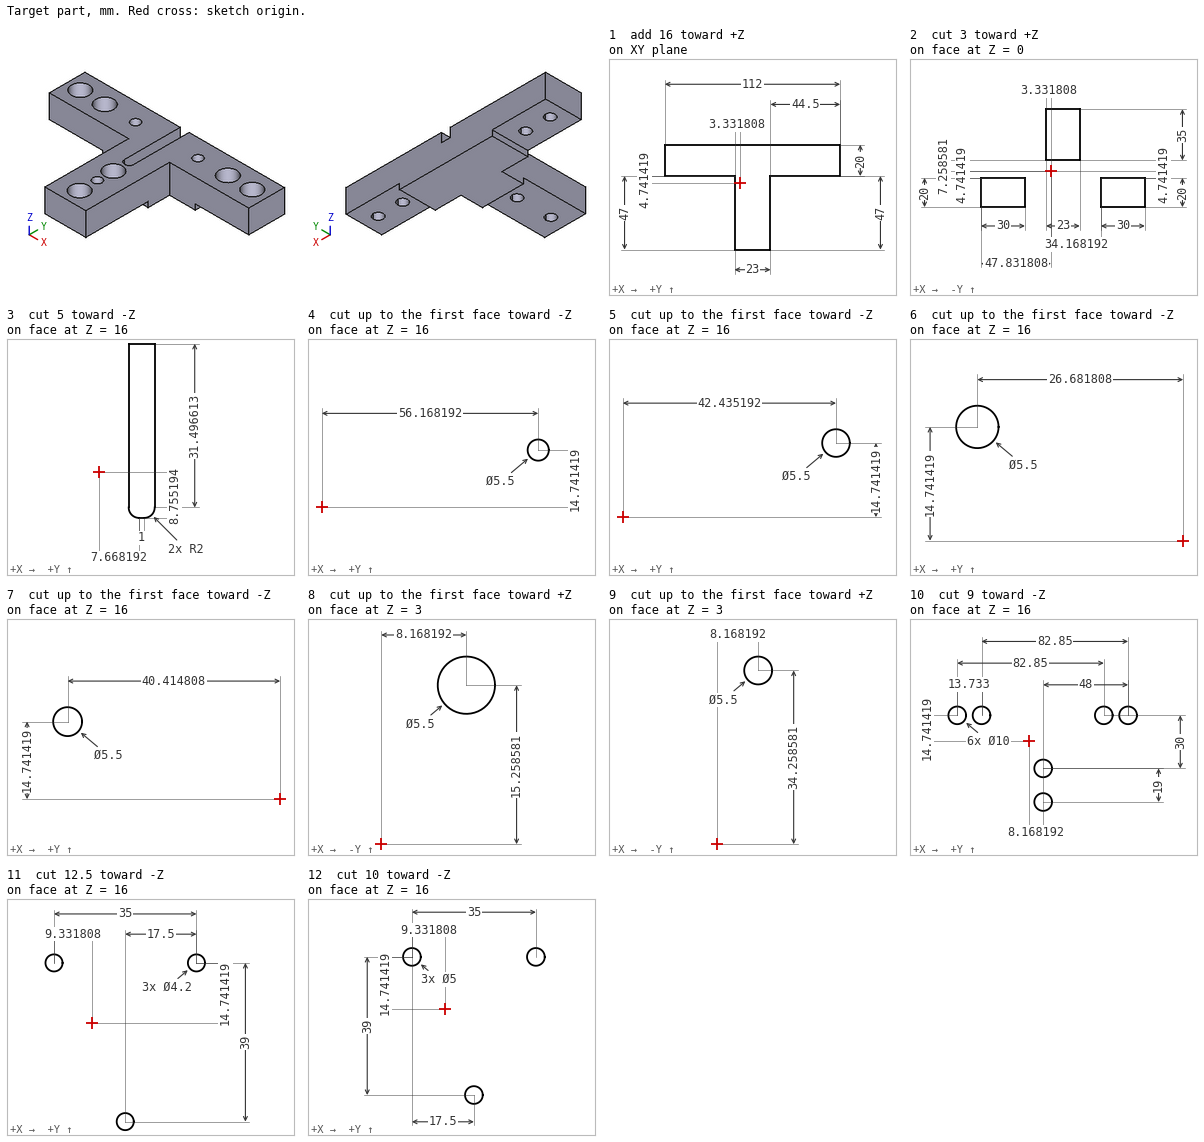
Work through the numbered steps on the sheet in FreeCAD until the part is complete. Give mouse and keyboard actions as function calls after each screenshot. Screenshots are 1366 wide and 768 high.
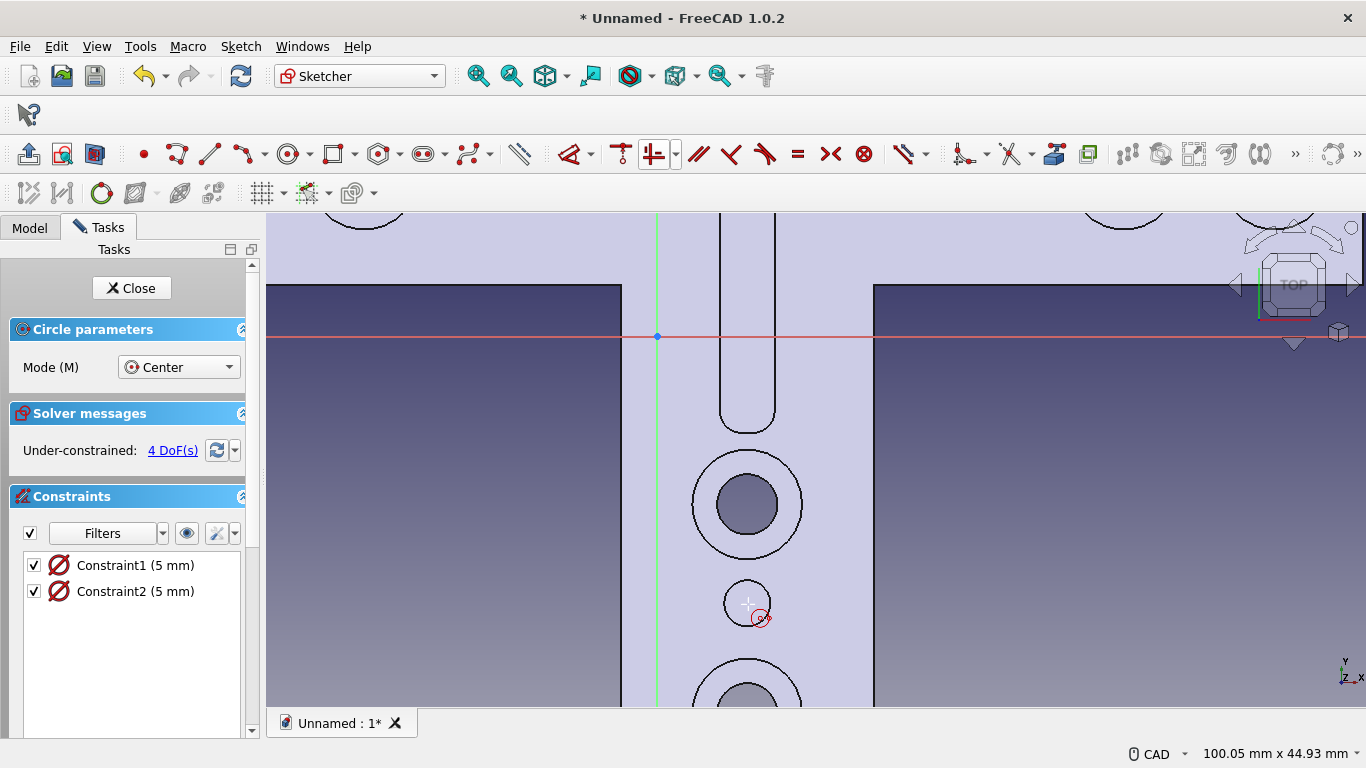
click(747, 603)
move(767, 584)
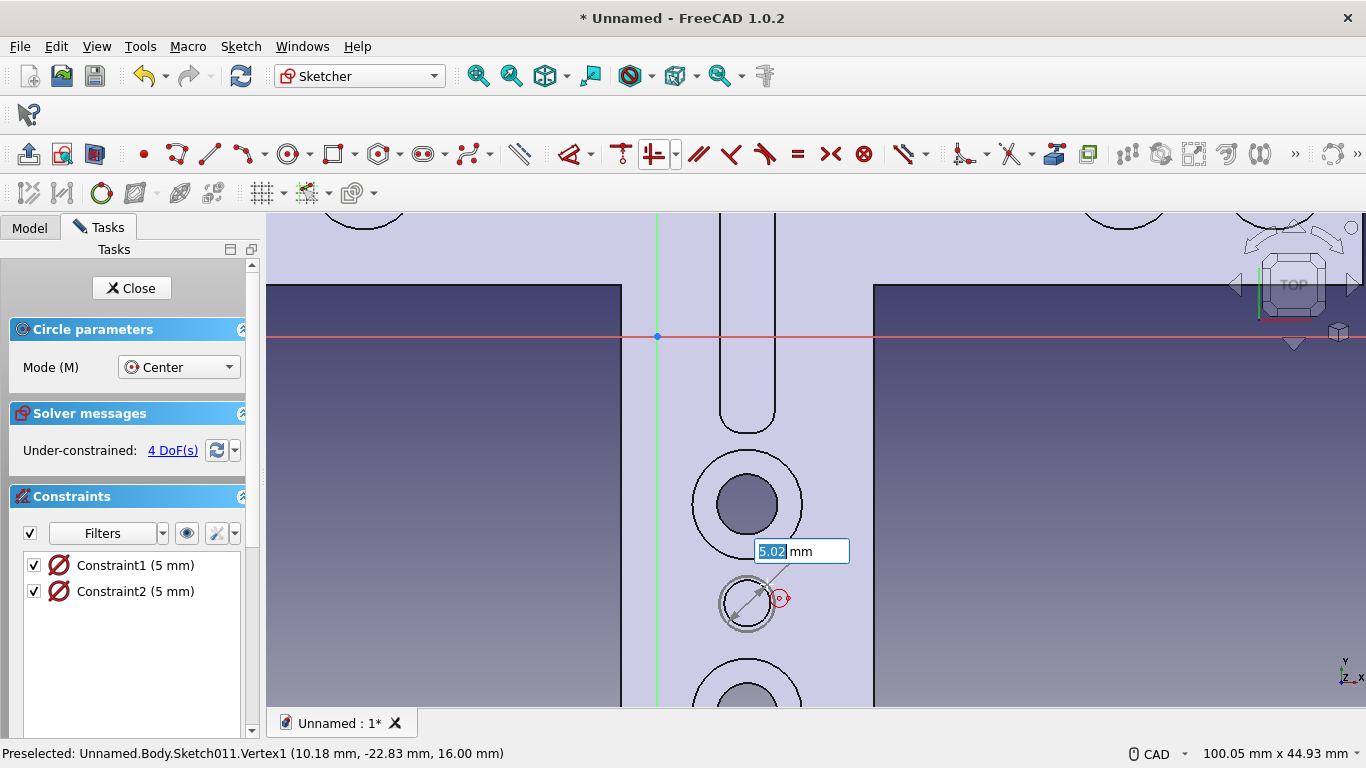
text(5)
key(Return)
key(Escape)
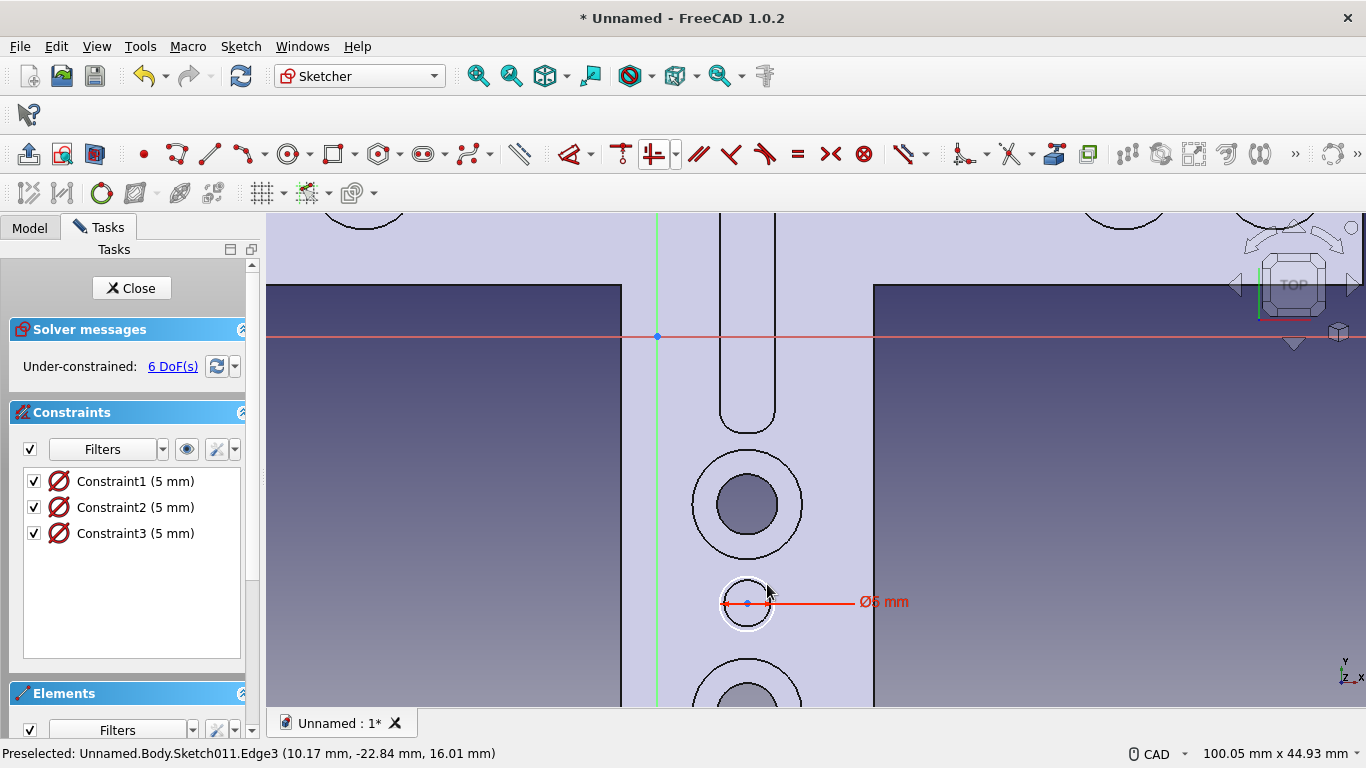
scroll(748, 604, down, 2)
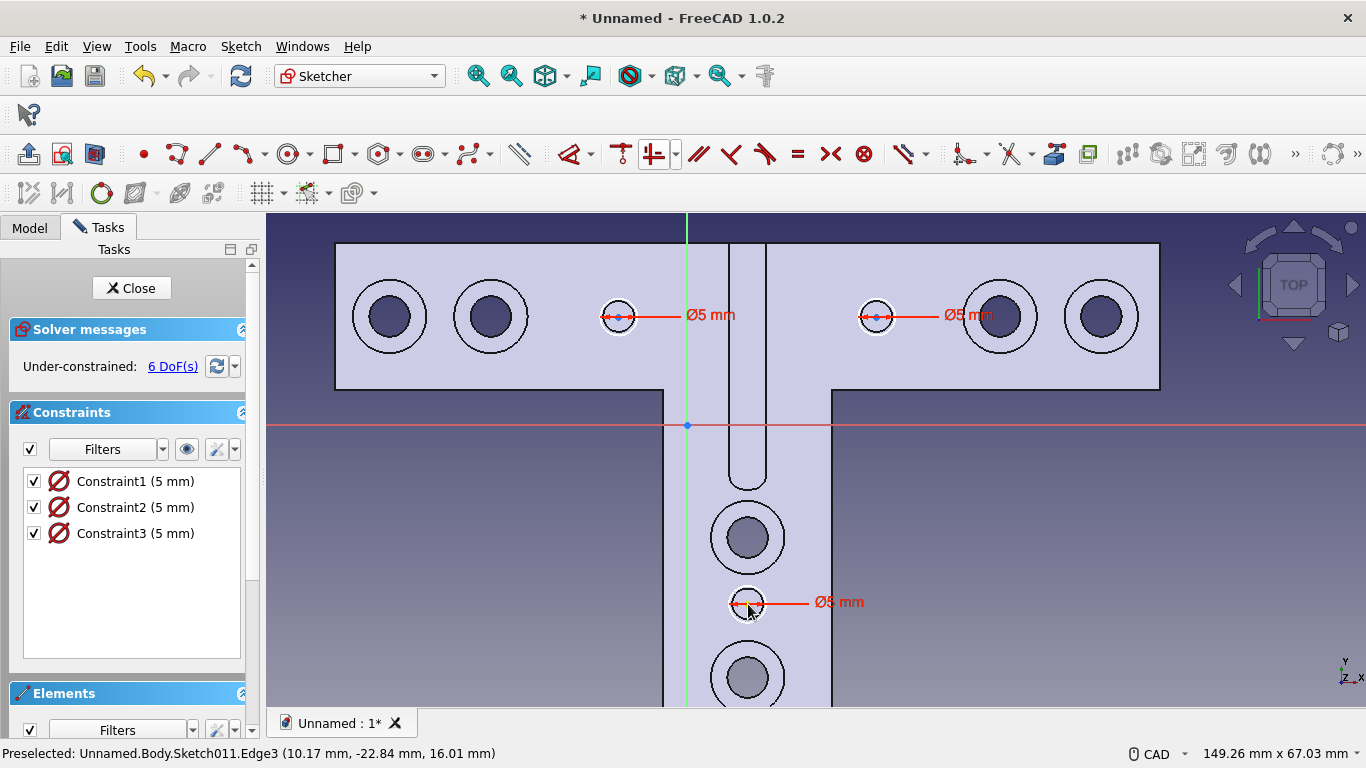
click(619, 317)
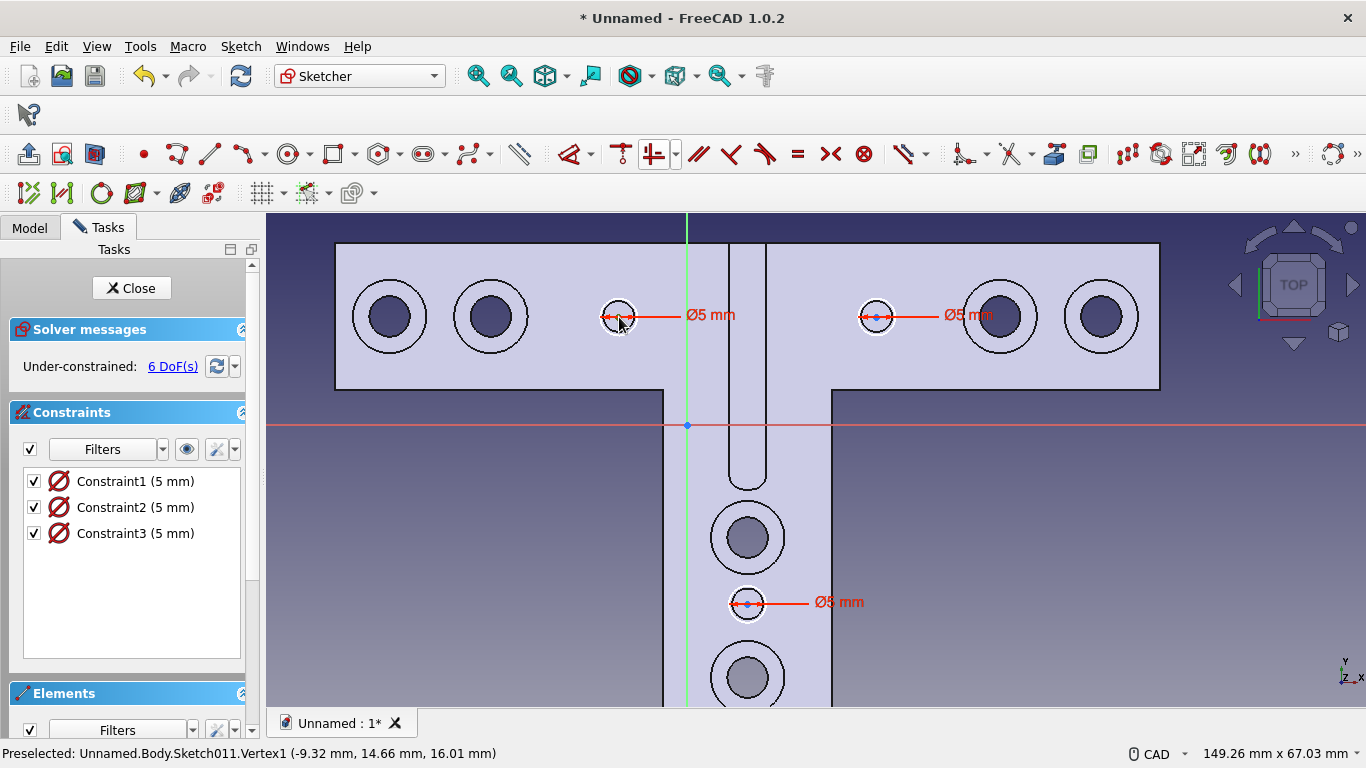
click(877, 317)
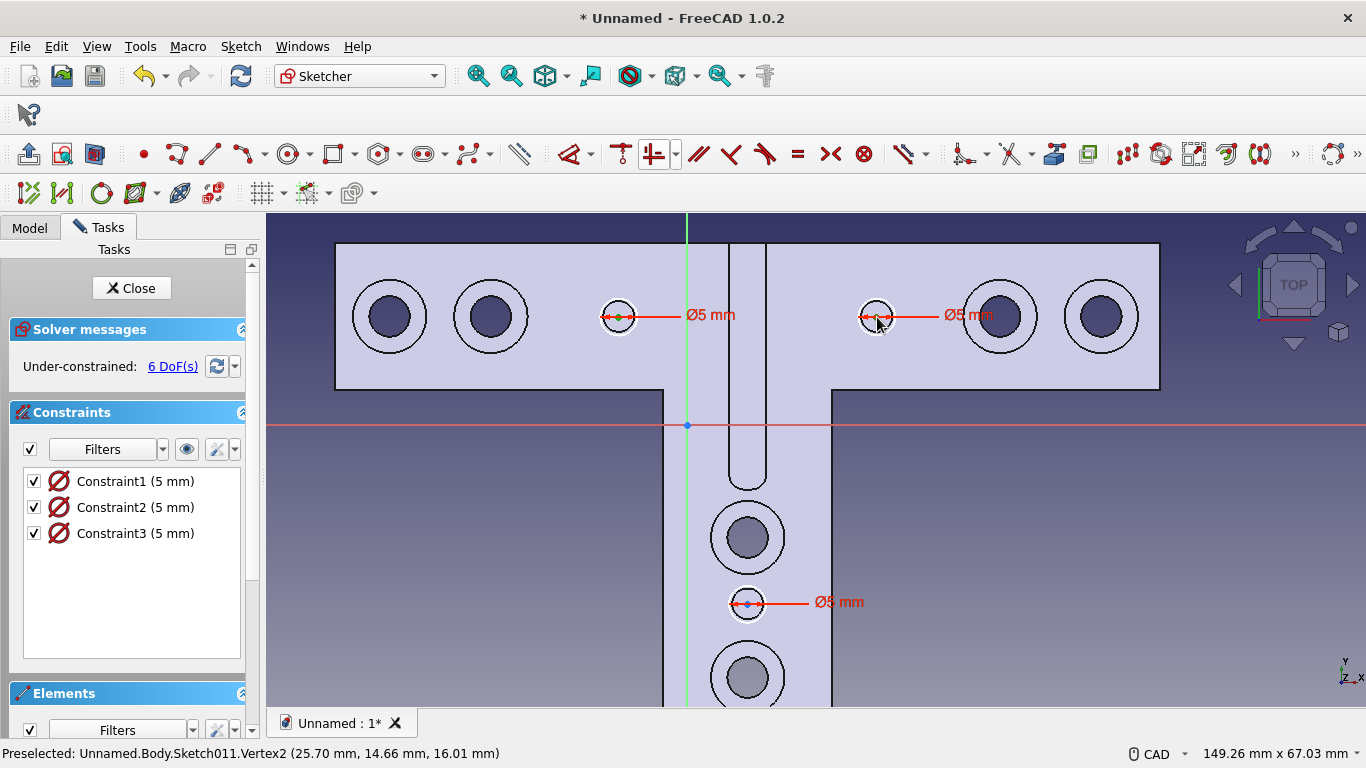
key(h)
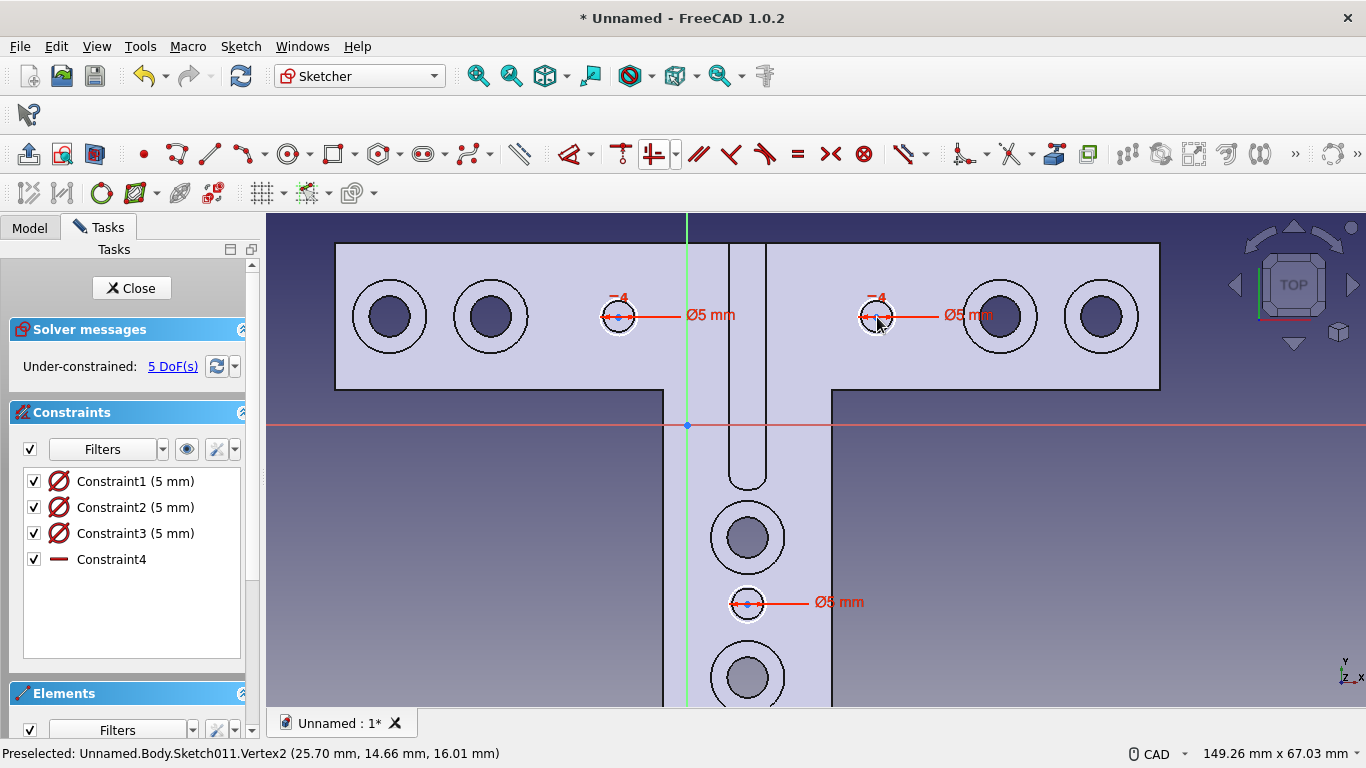
click(568, 154)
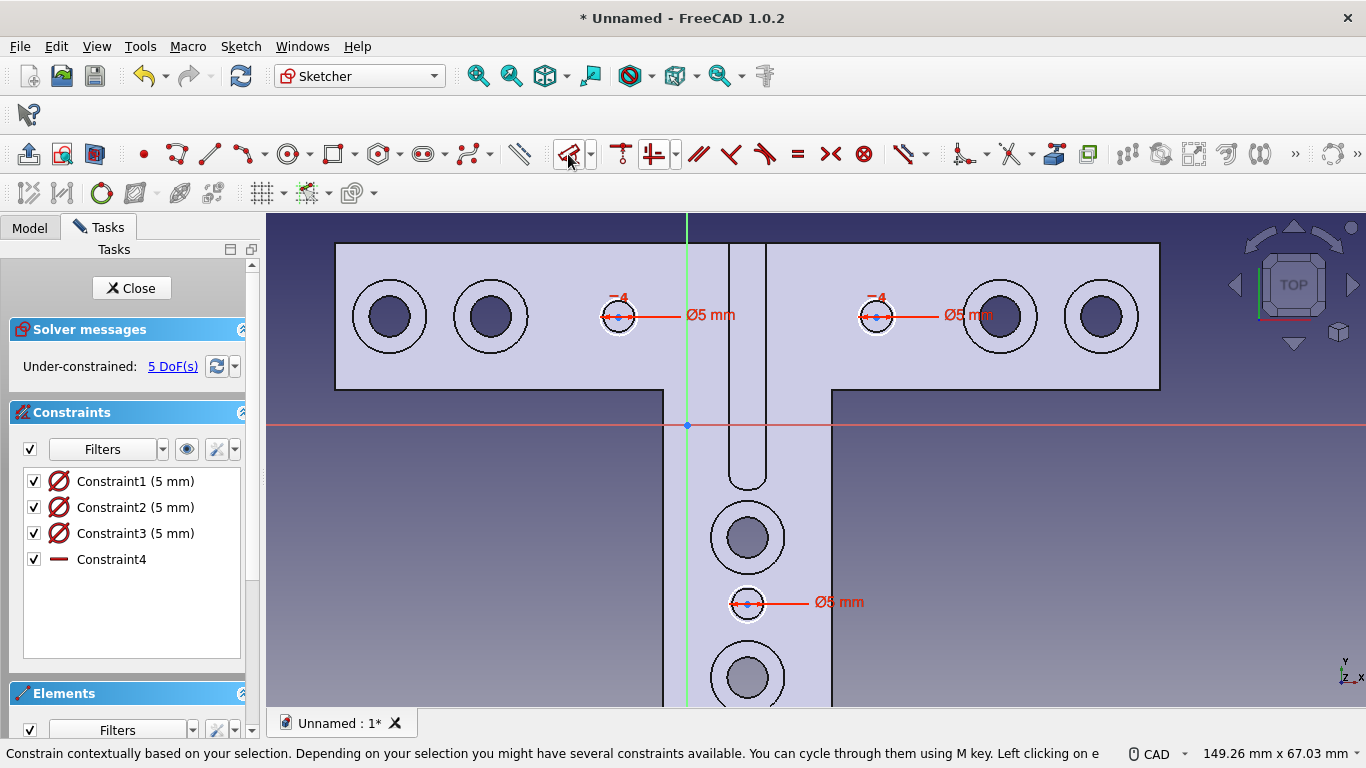
click(619, 317)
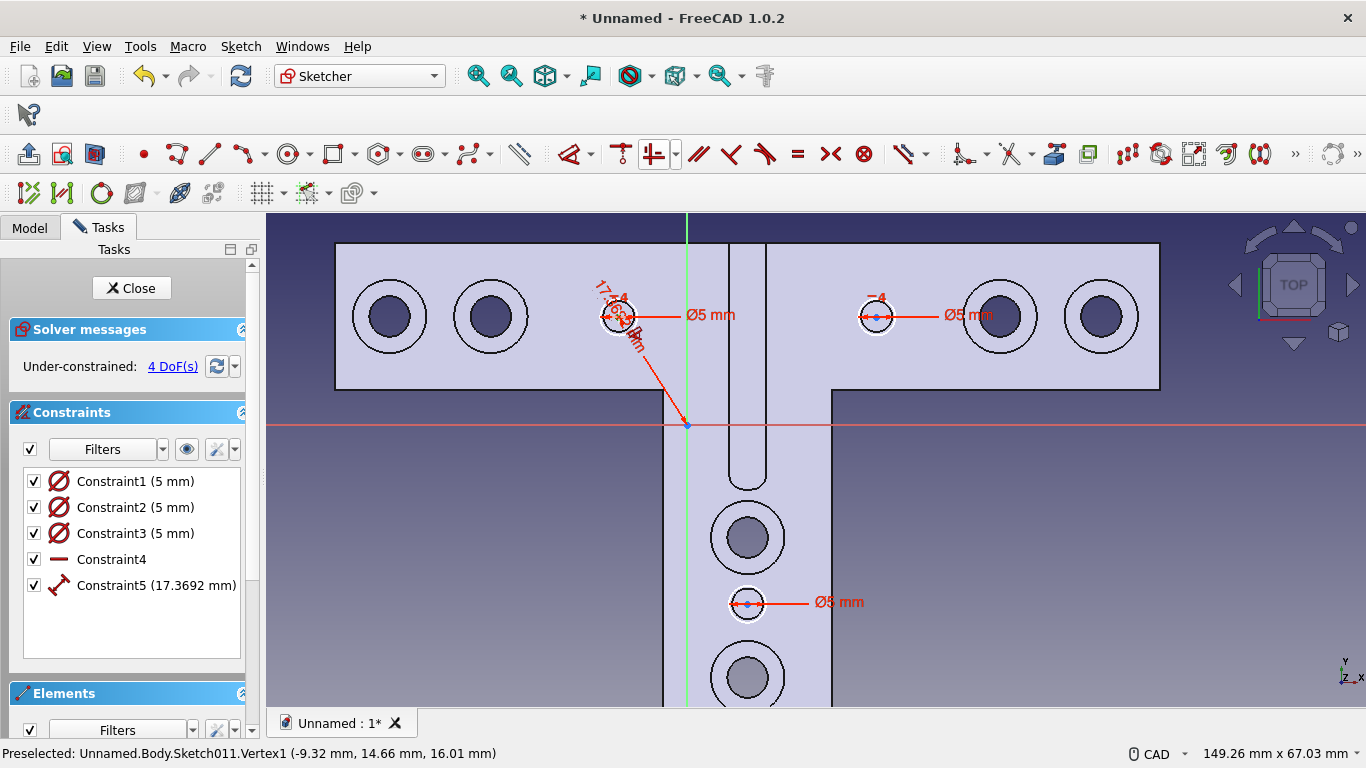
click(877, 317)
click(748, 283)